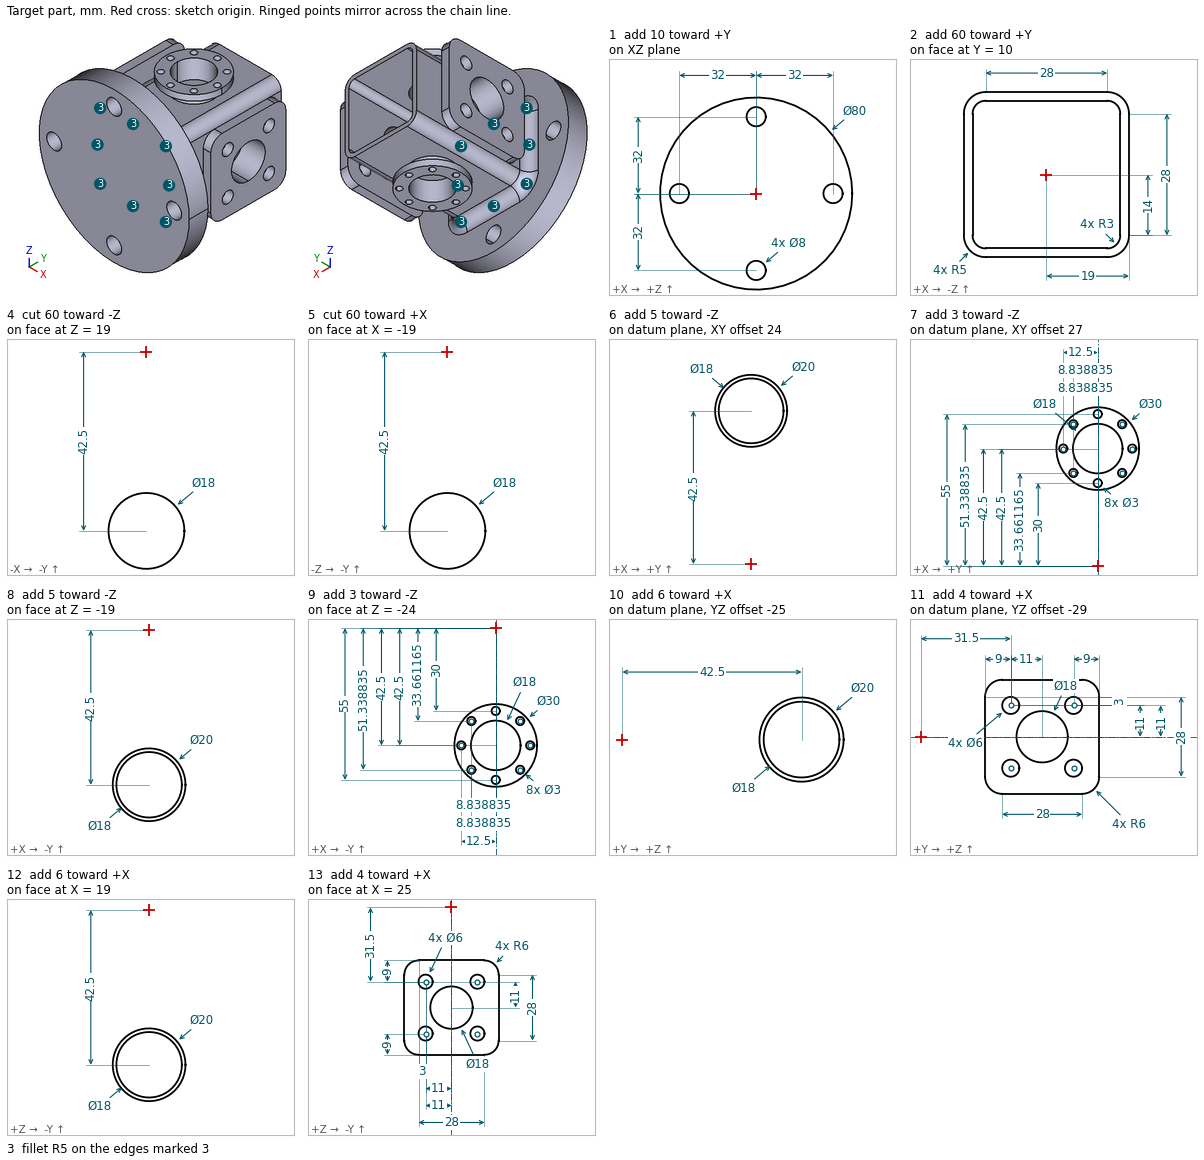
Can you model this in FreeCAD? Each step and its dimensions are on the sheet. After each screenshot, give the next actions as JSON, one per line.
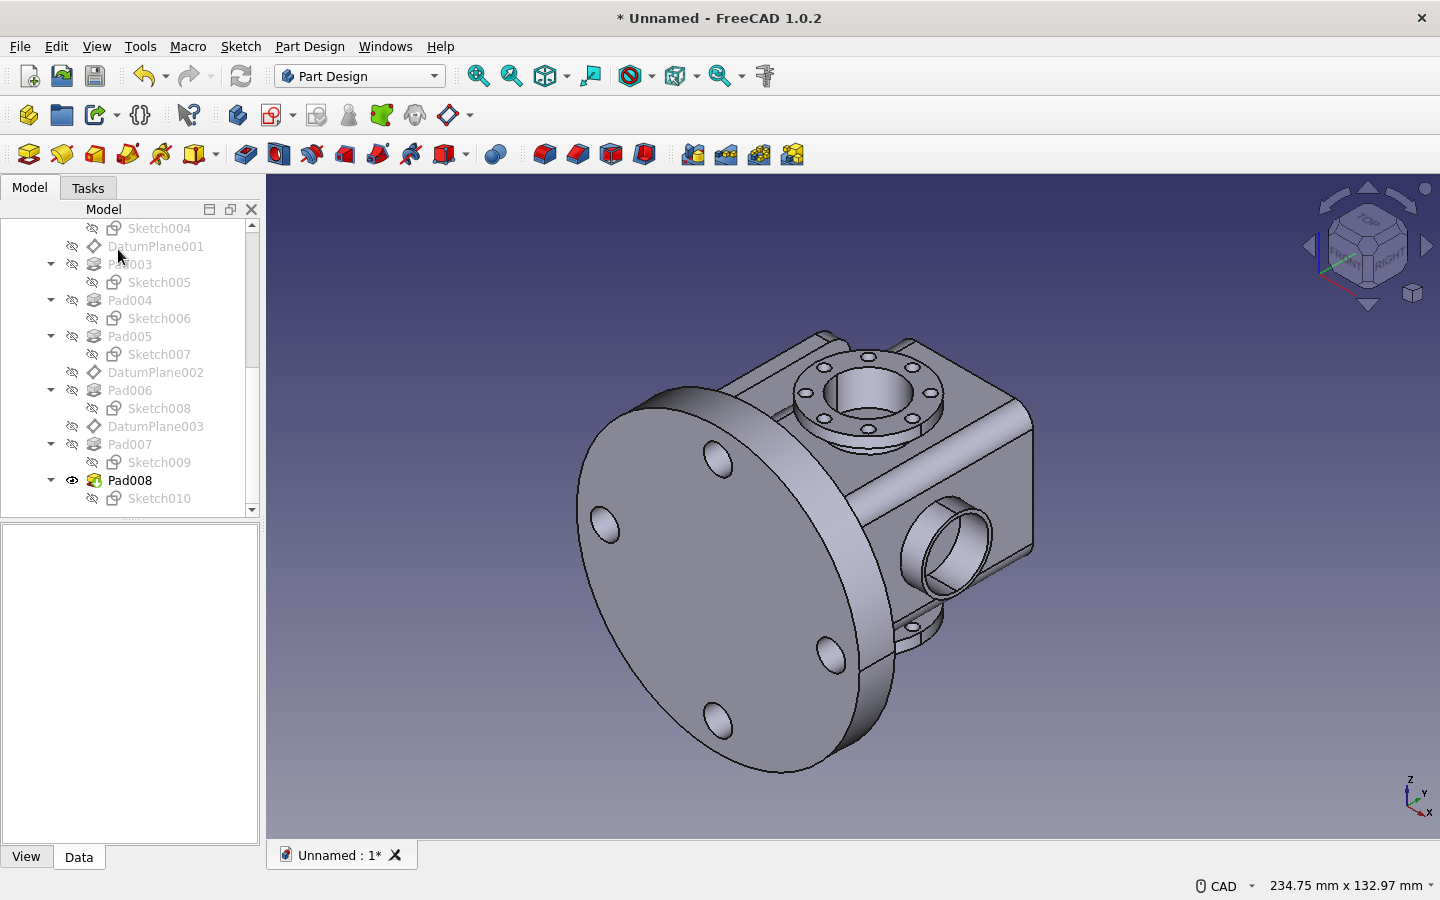
{"action": "scroll", "coordinate": [987, 524], "scroll_direction": "up", "scroll_amount": 15}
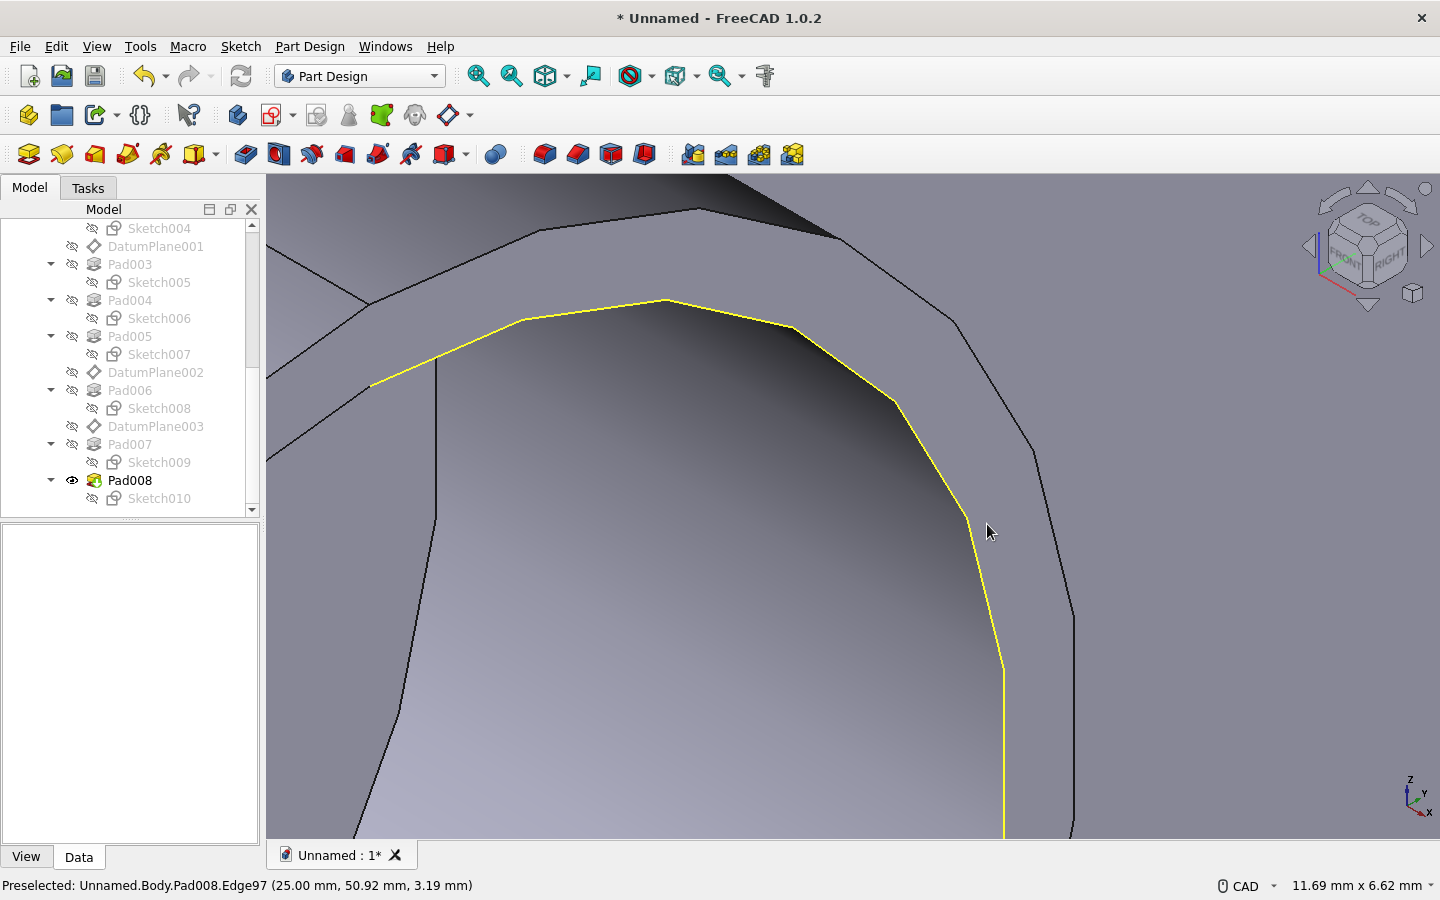
{"action": "left_click", "coordinate": [572, 304]}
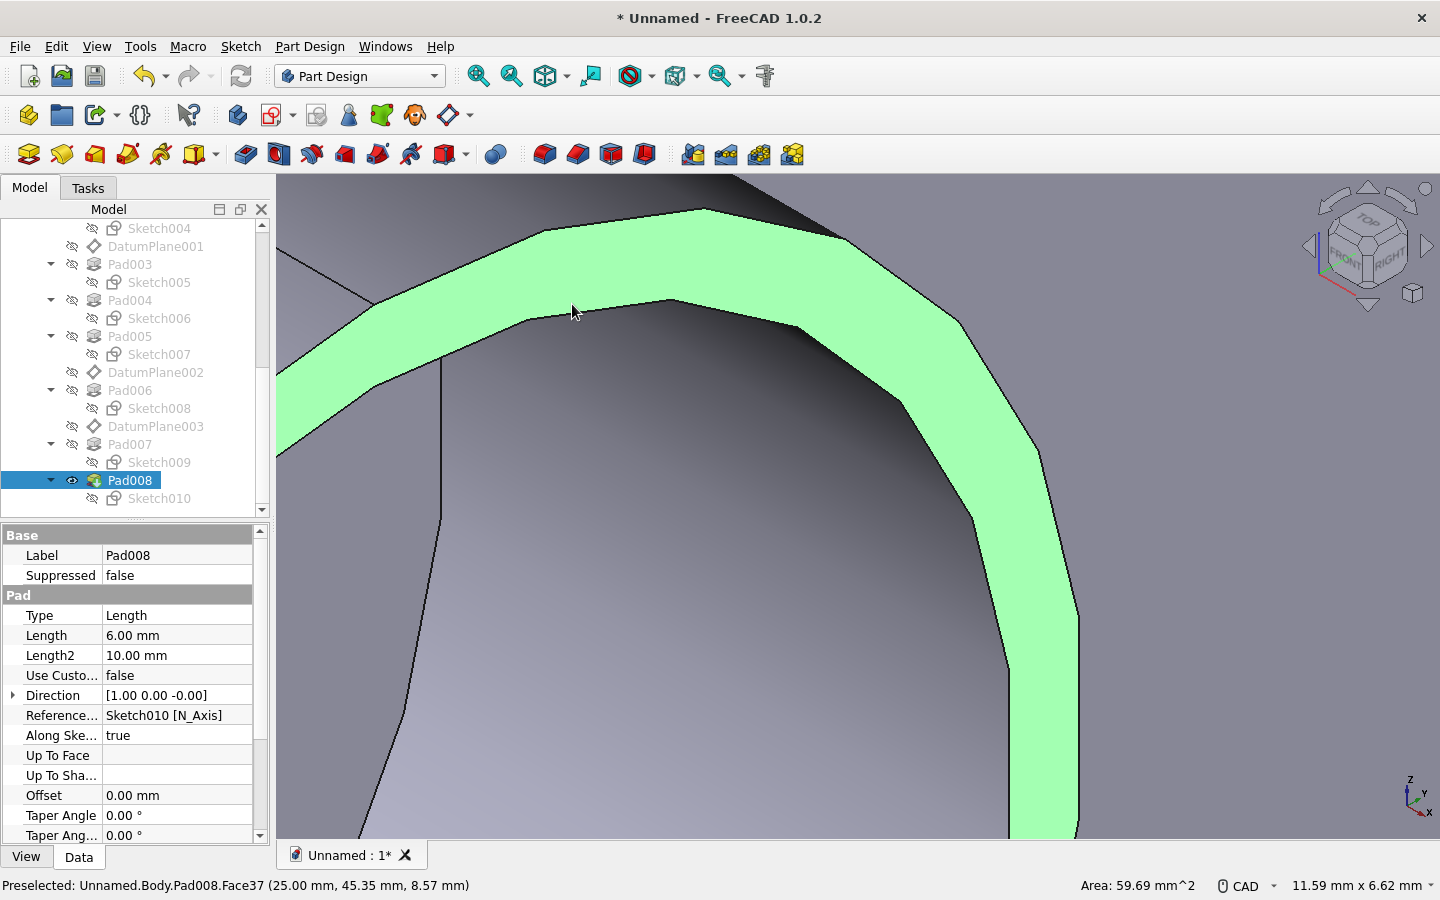
{"action": "left_click", "coordinate": [270, 116]}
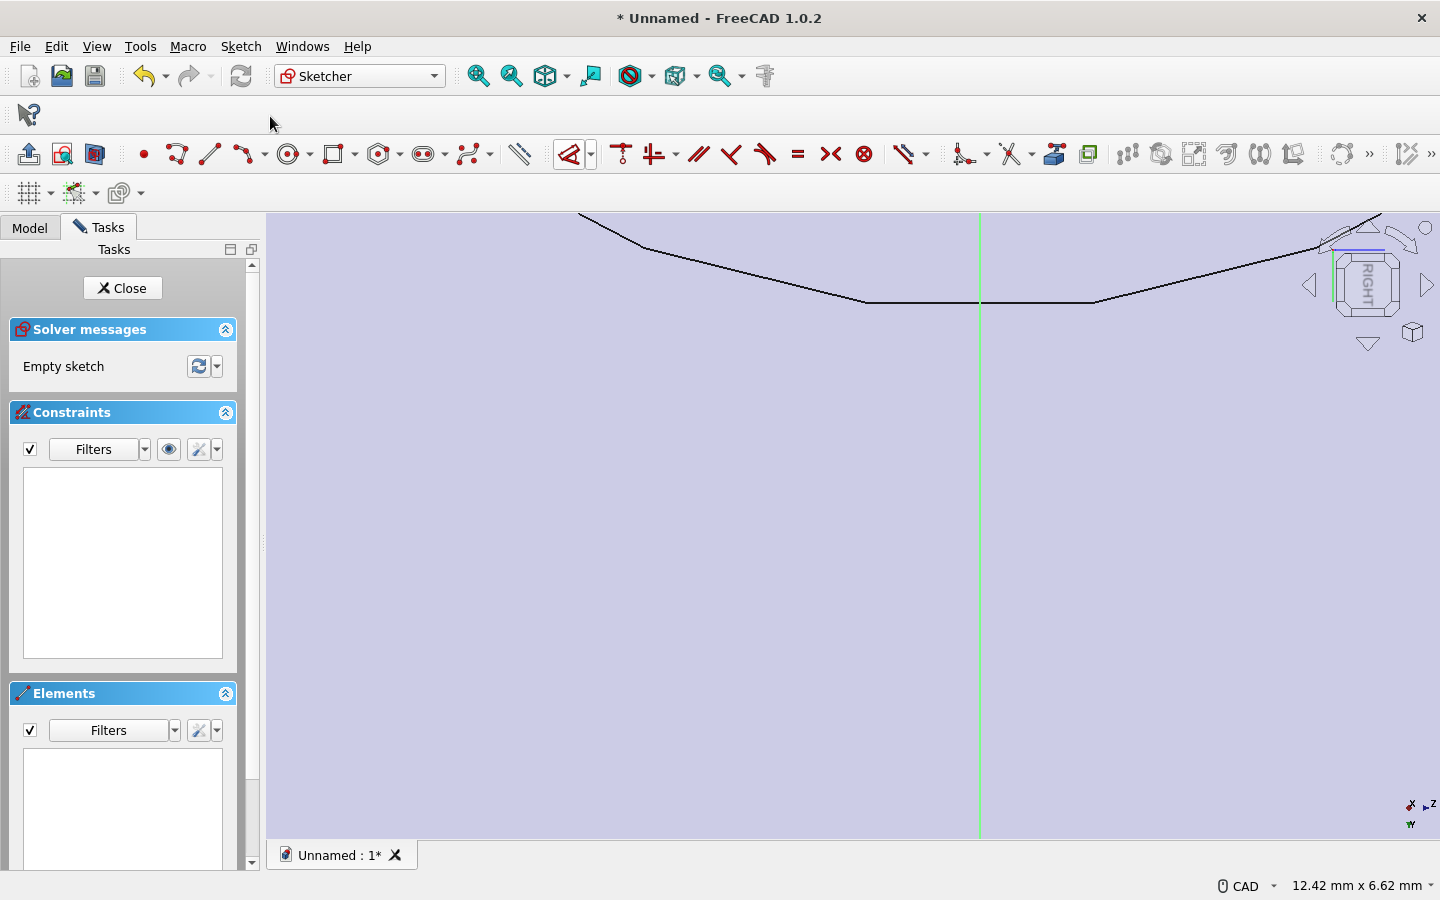
{"action": "scroll", "coordinate": [769, 705], "scroll_direction": "down", "scroll_amount": 13}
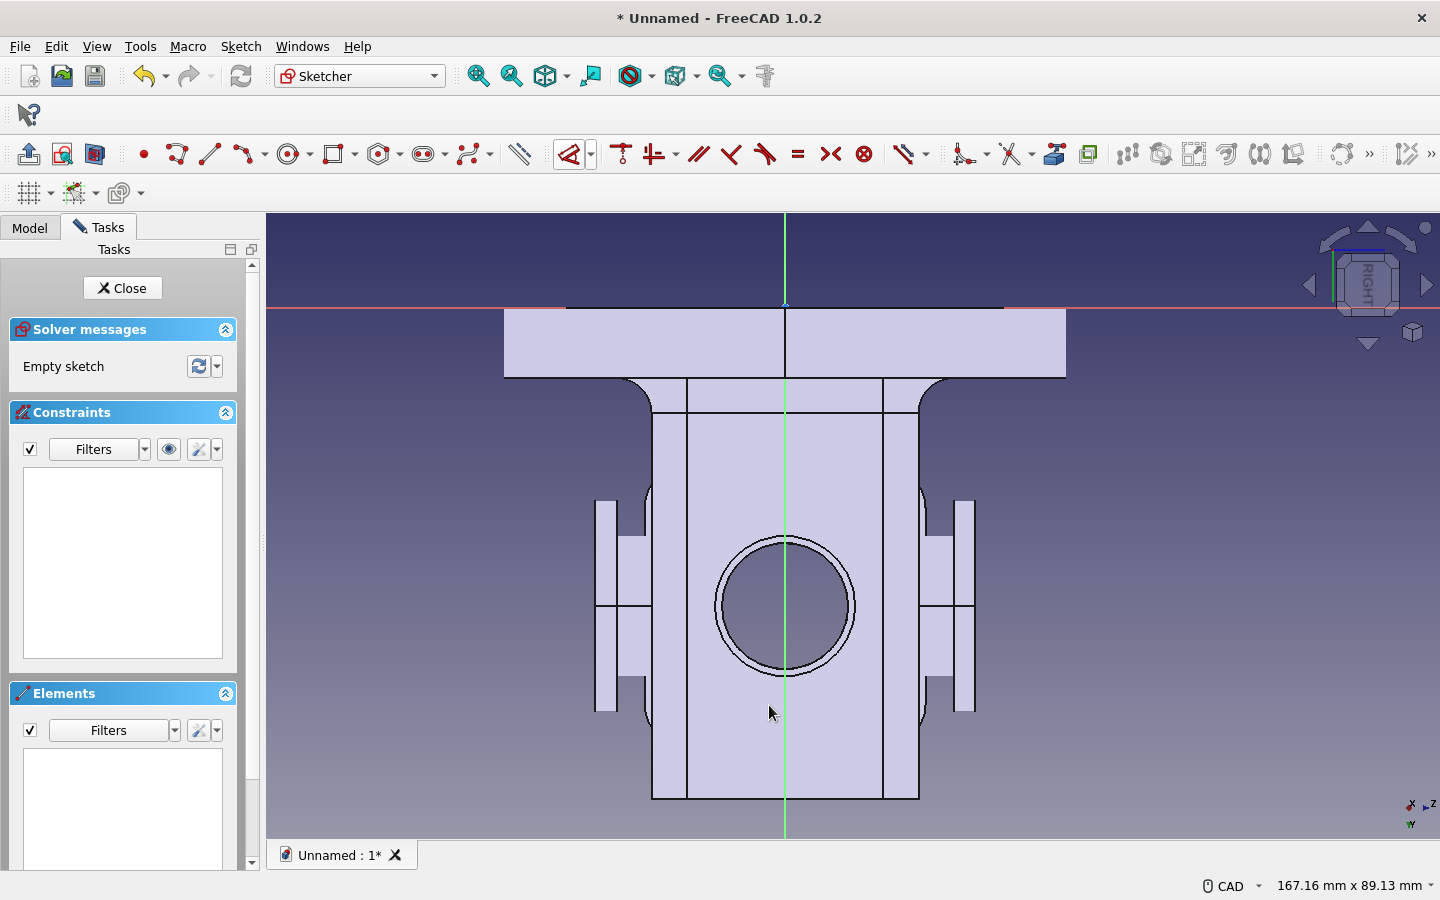
{"action": "key", "text": "g l"}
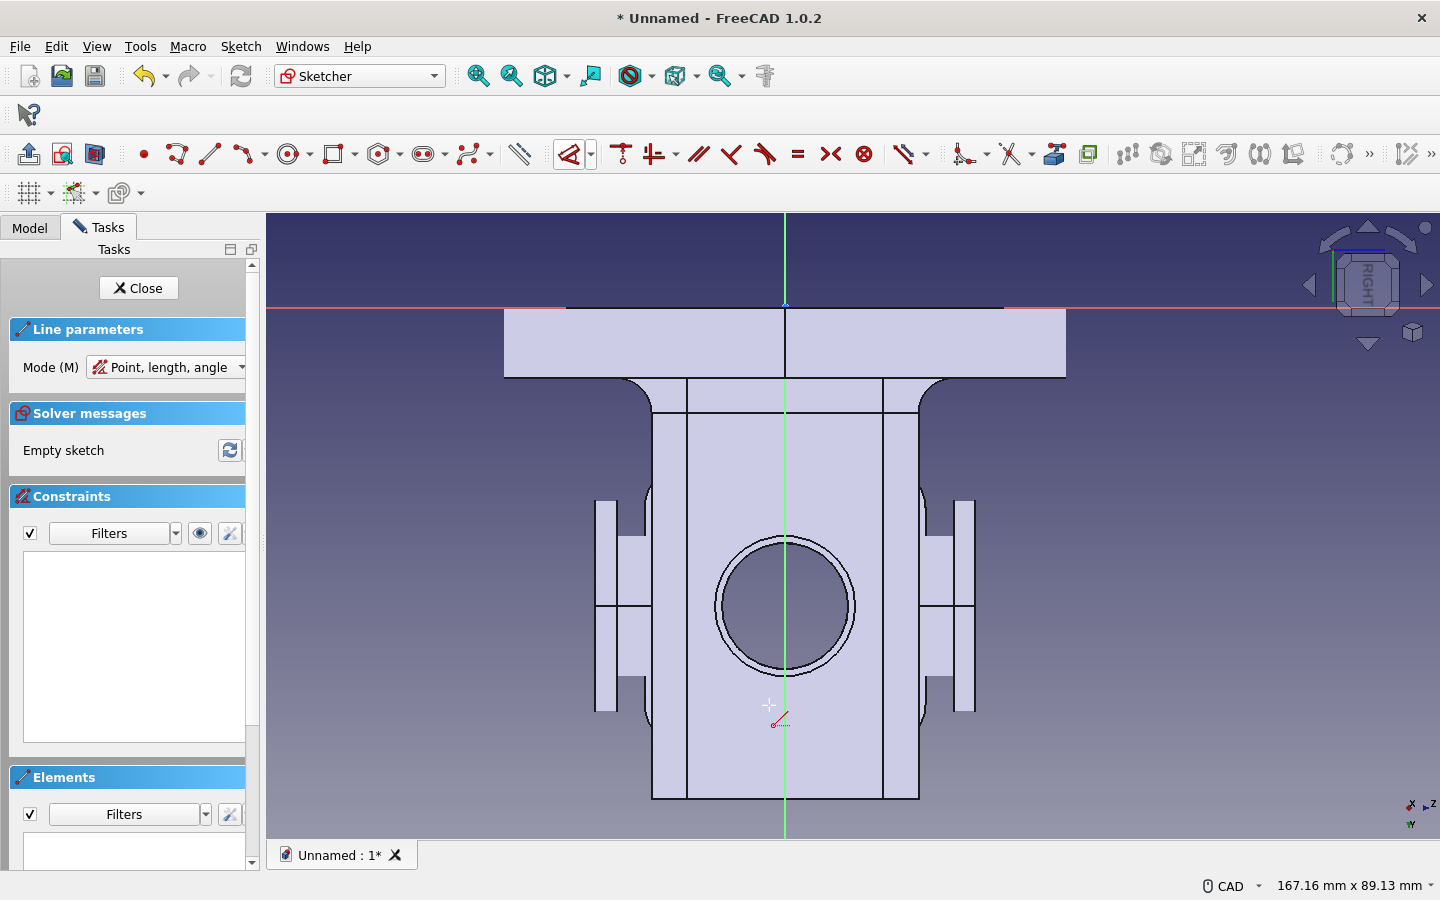
{"action": "left_click", "coordinate": [687, 747]}
{"action": "left_click", "coordinate": [883, 747]}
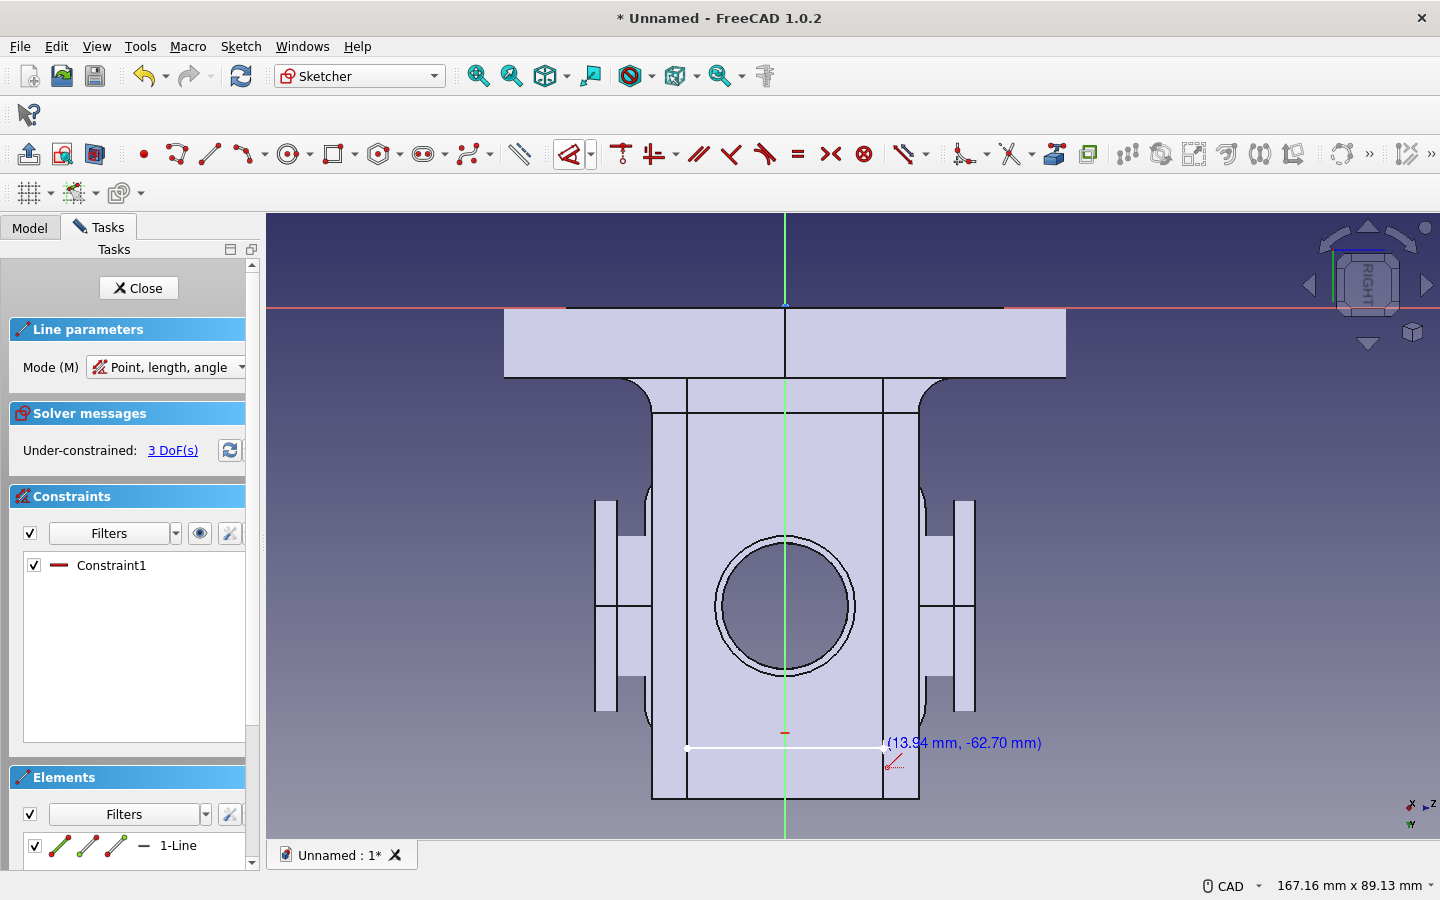
{"action": "left_click", "coordinate": [926, 704]}
{"action": "left_click", "coordinate": [926, 508]}